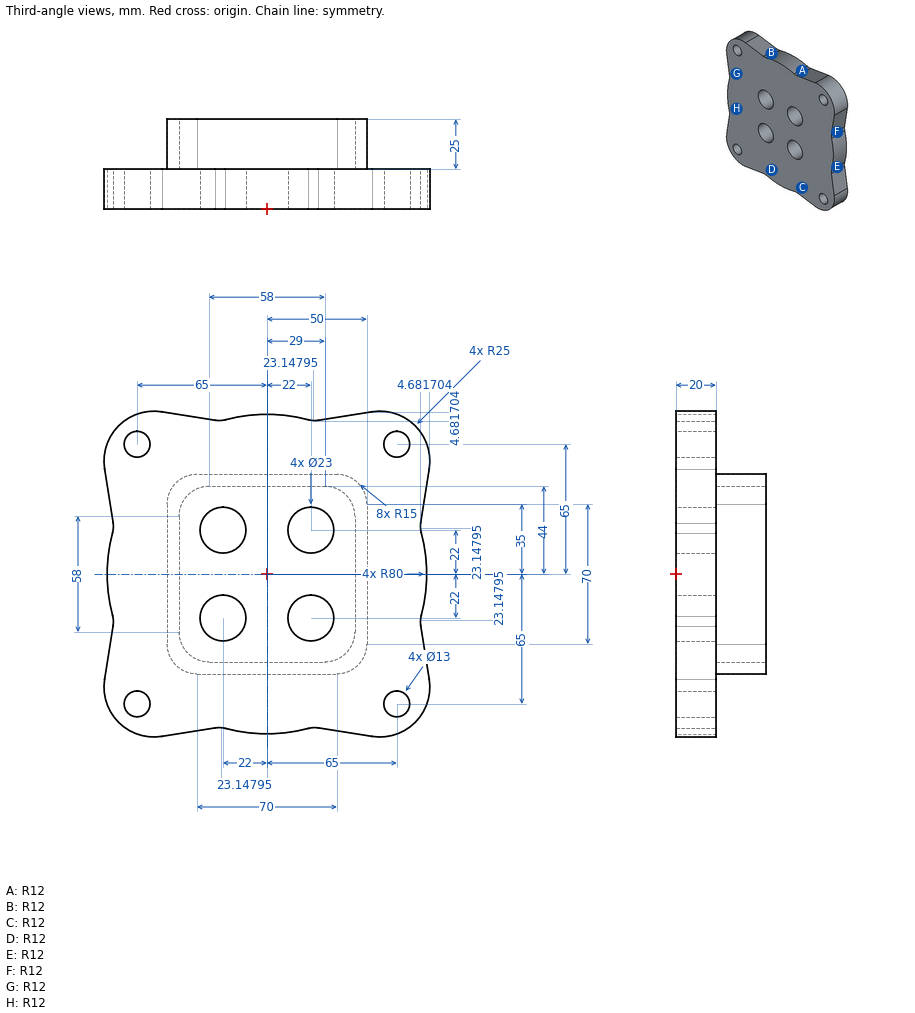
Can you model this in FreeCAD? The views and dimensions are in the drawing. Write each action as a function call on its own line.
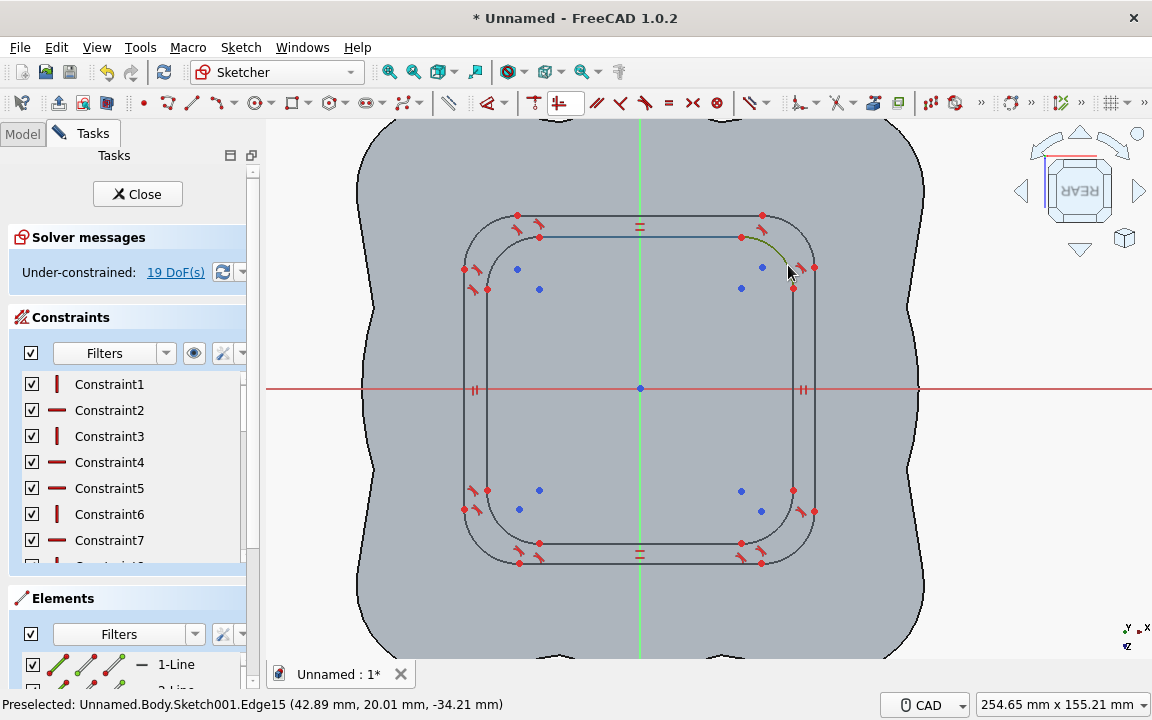
click(646, 104)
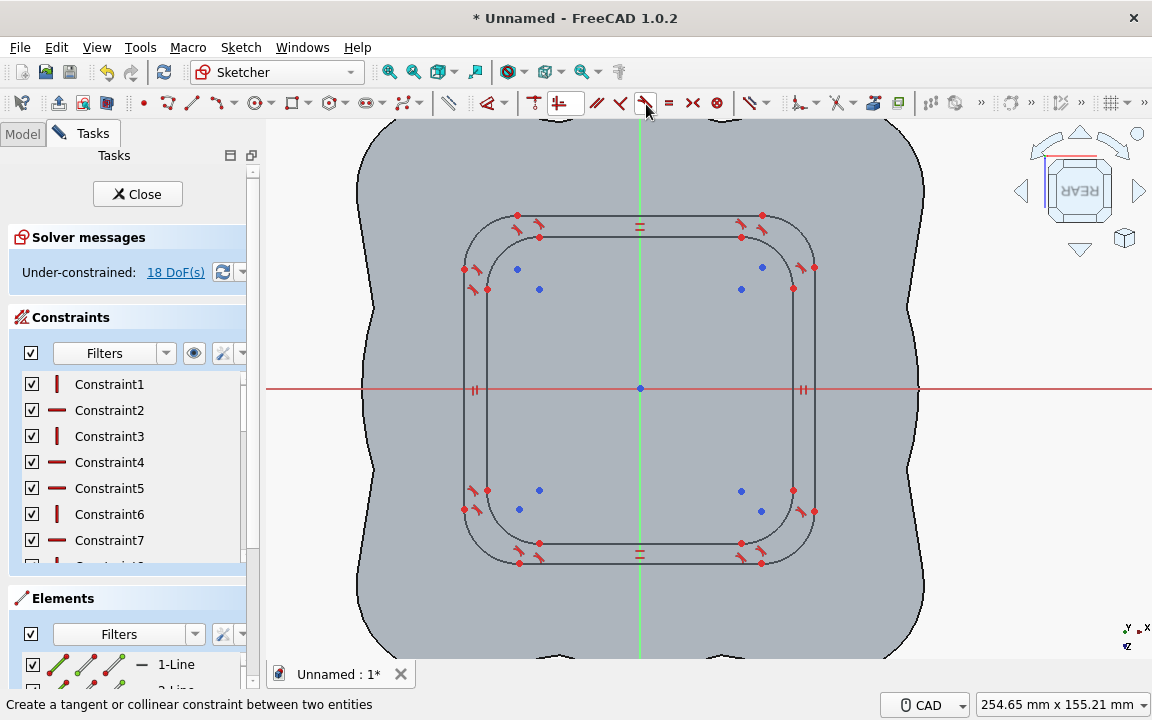
click(793, 350)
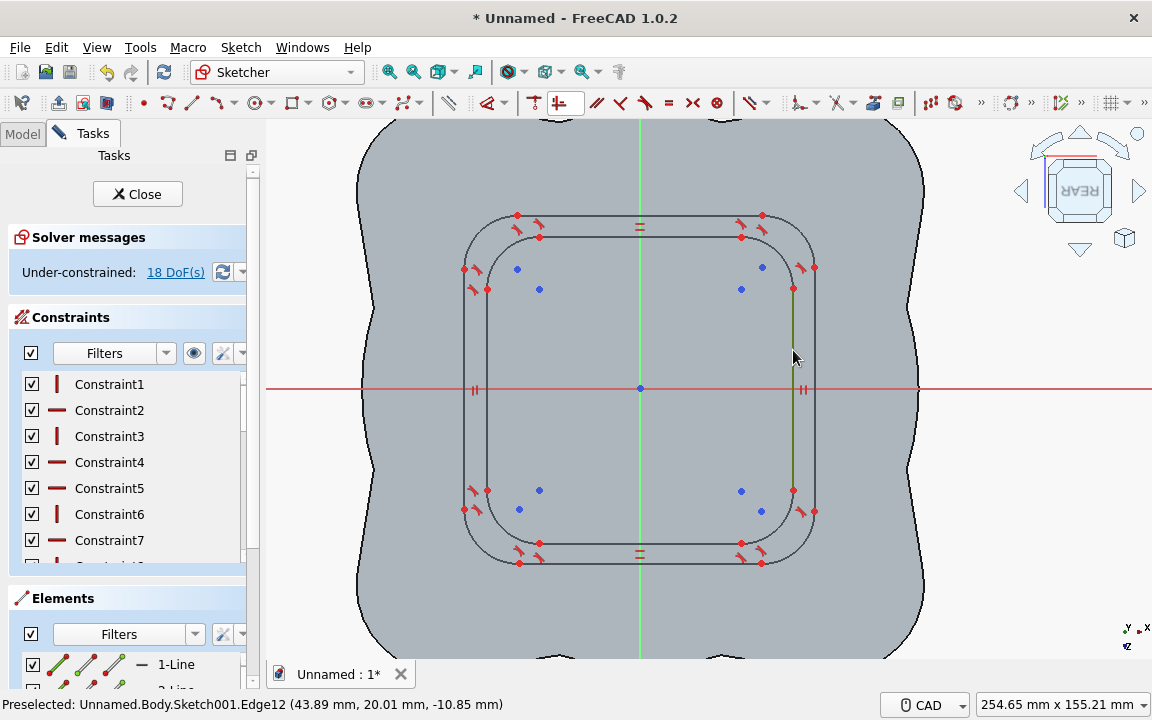
click(787, 265)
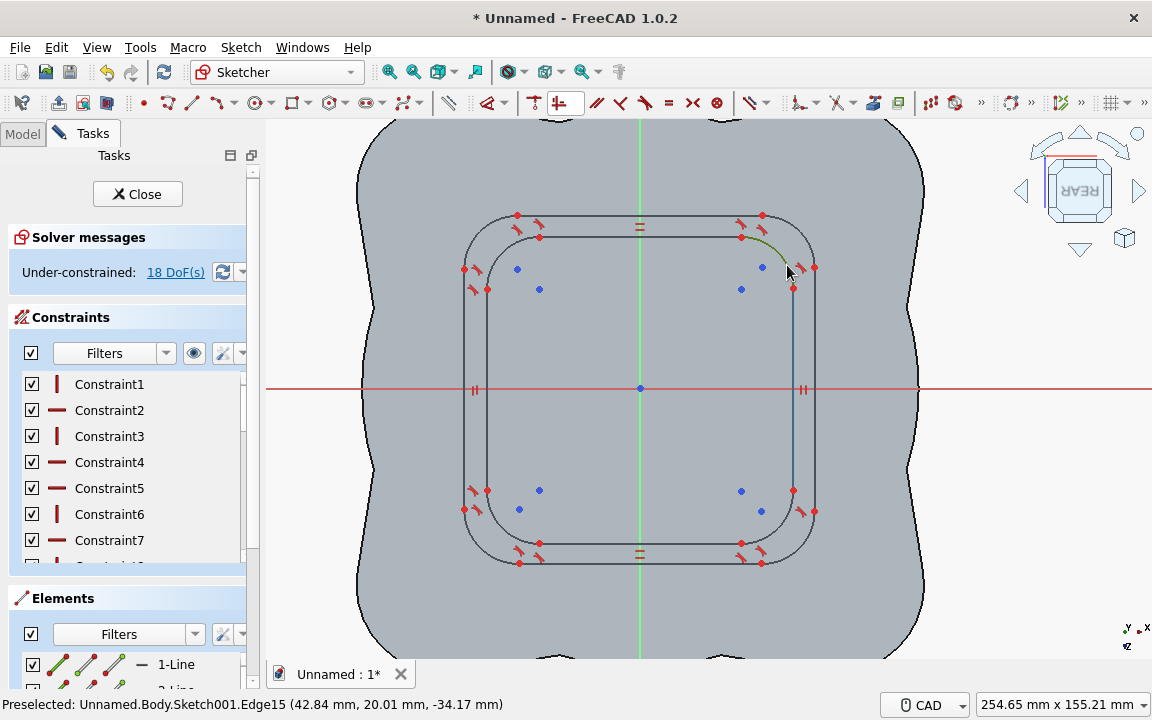
click(646, 104)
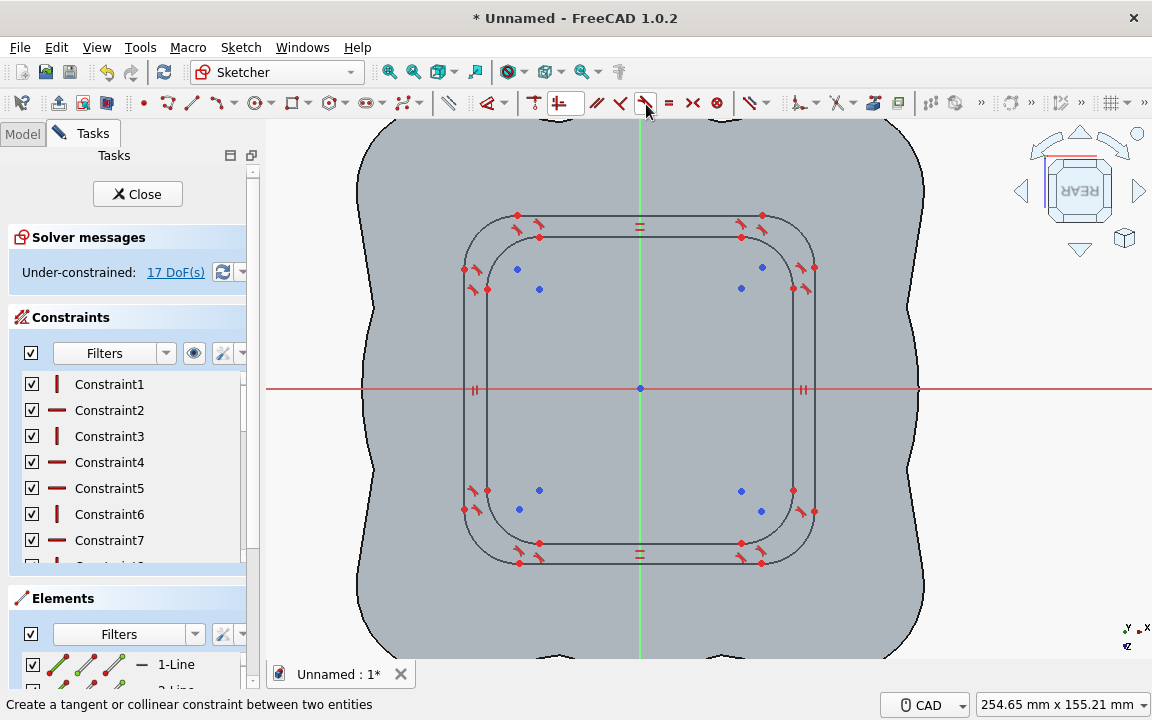
click(793, 350)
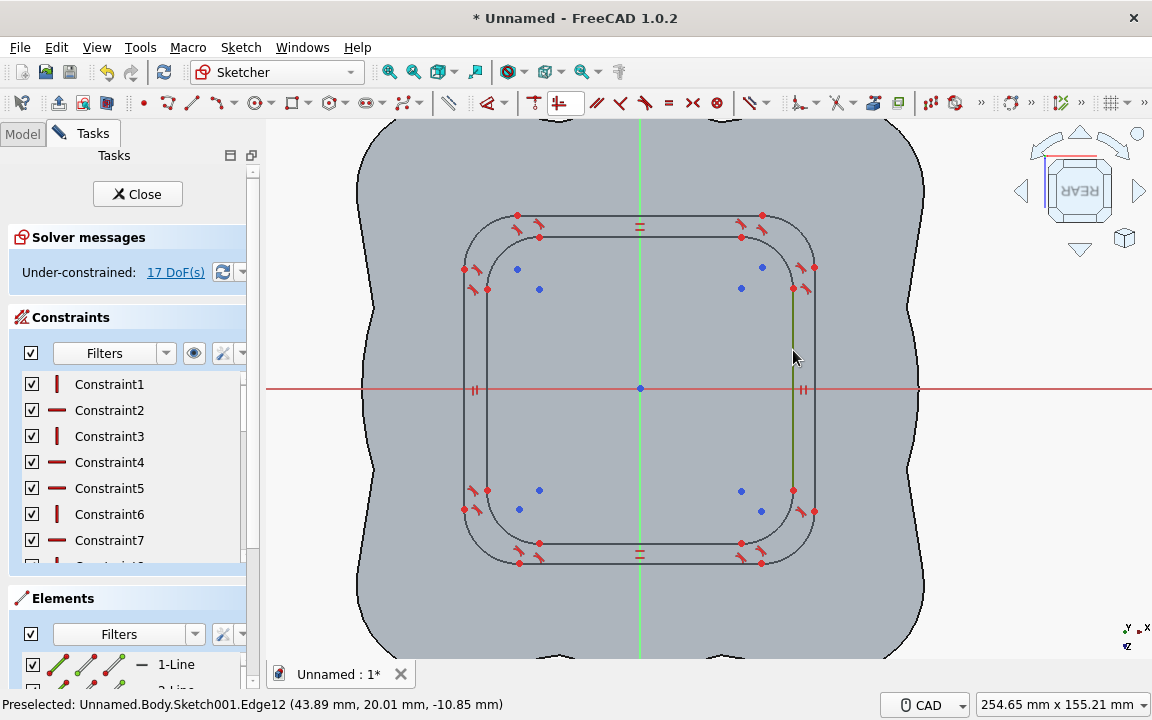
click(765, 538)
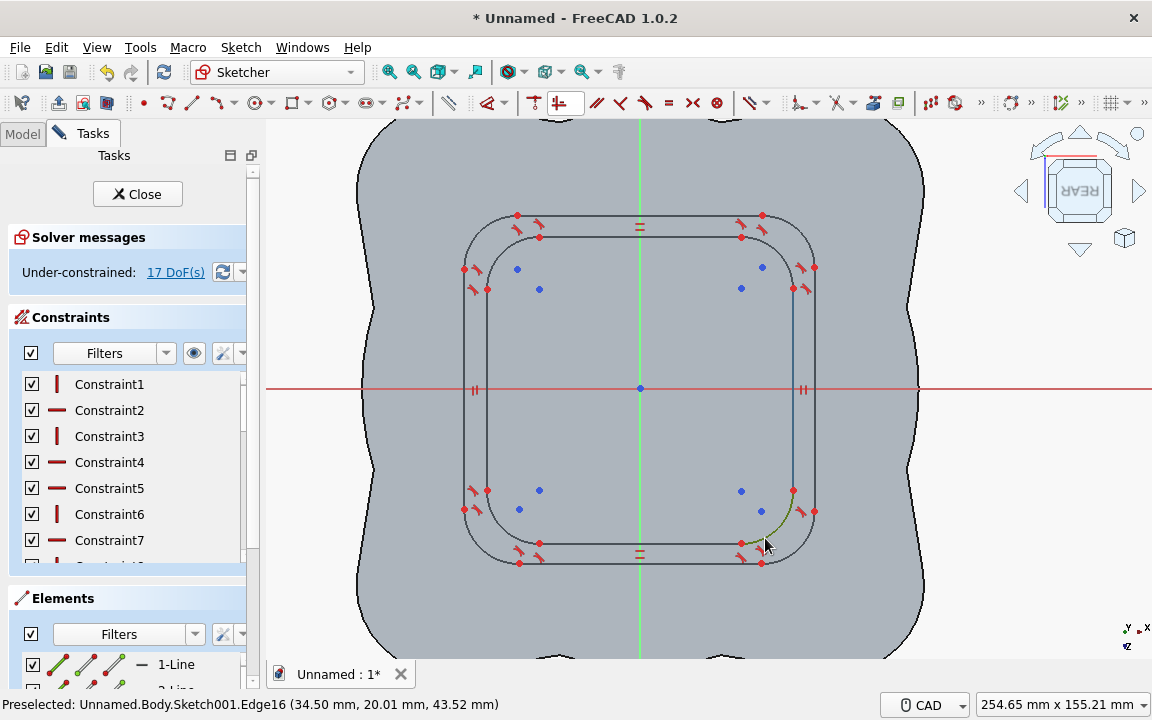
click(646, 104)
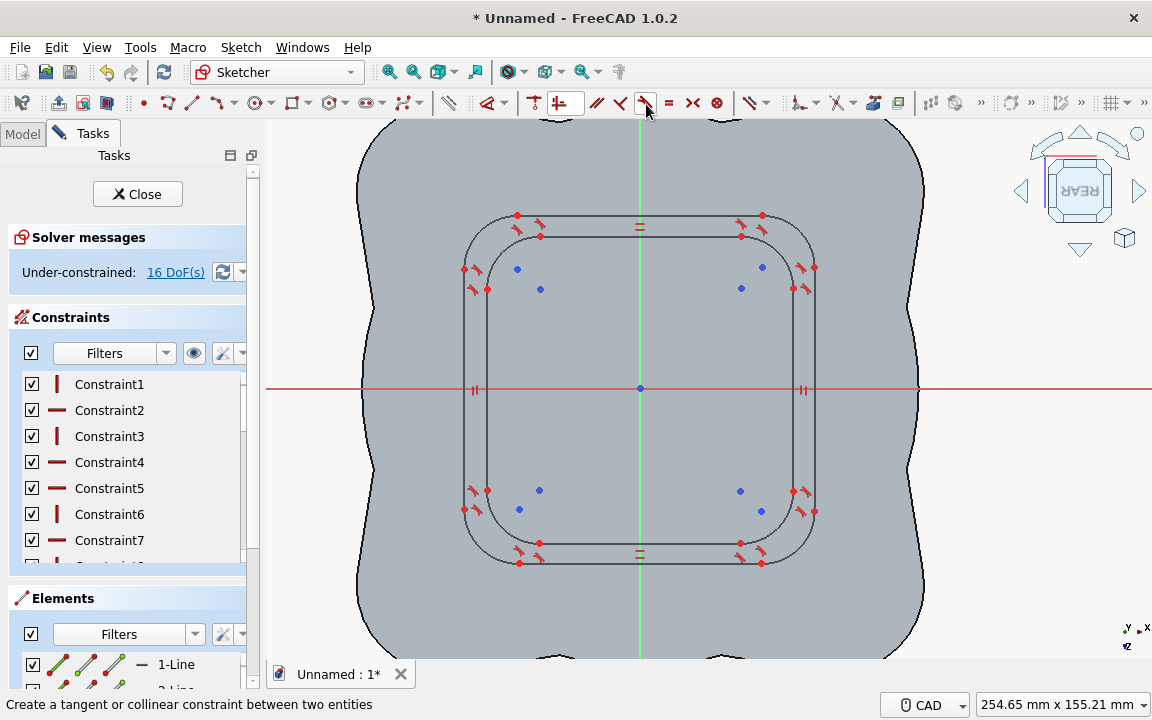
click(809, 244)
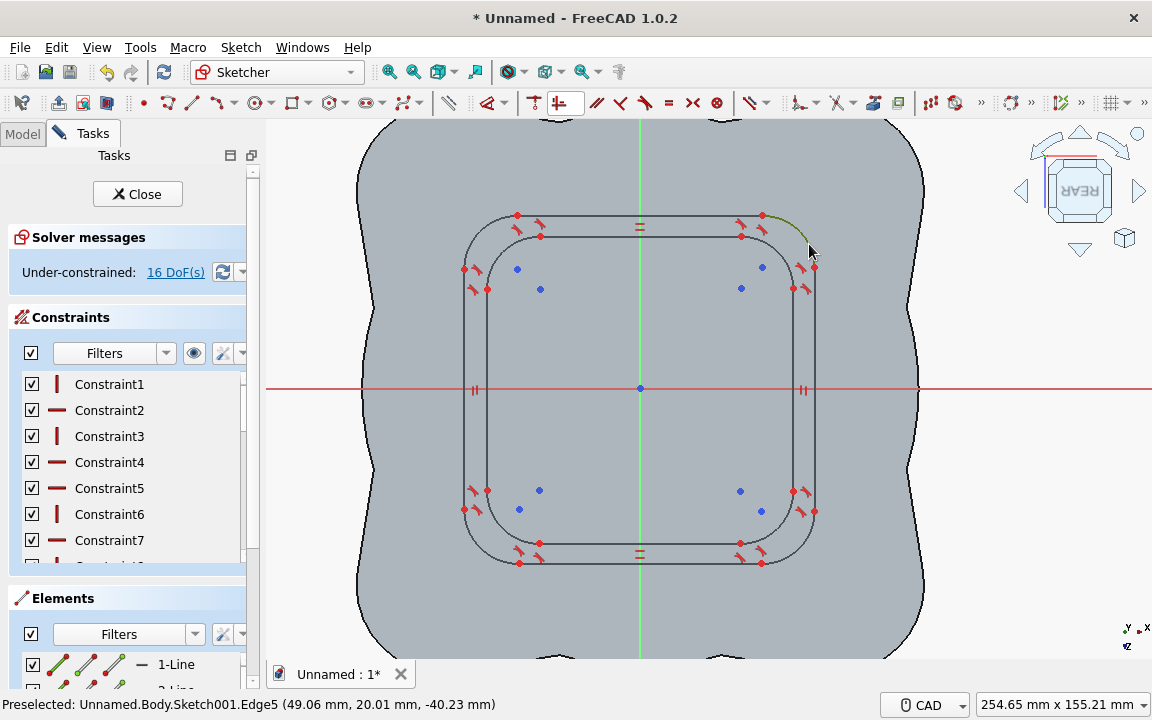
click(494, 222)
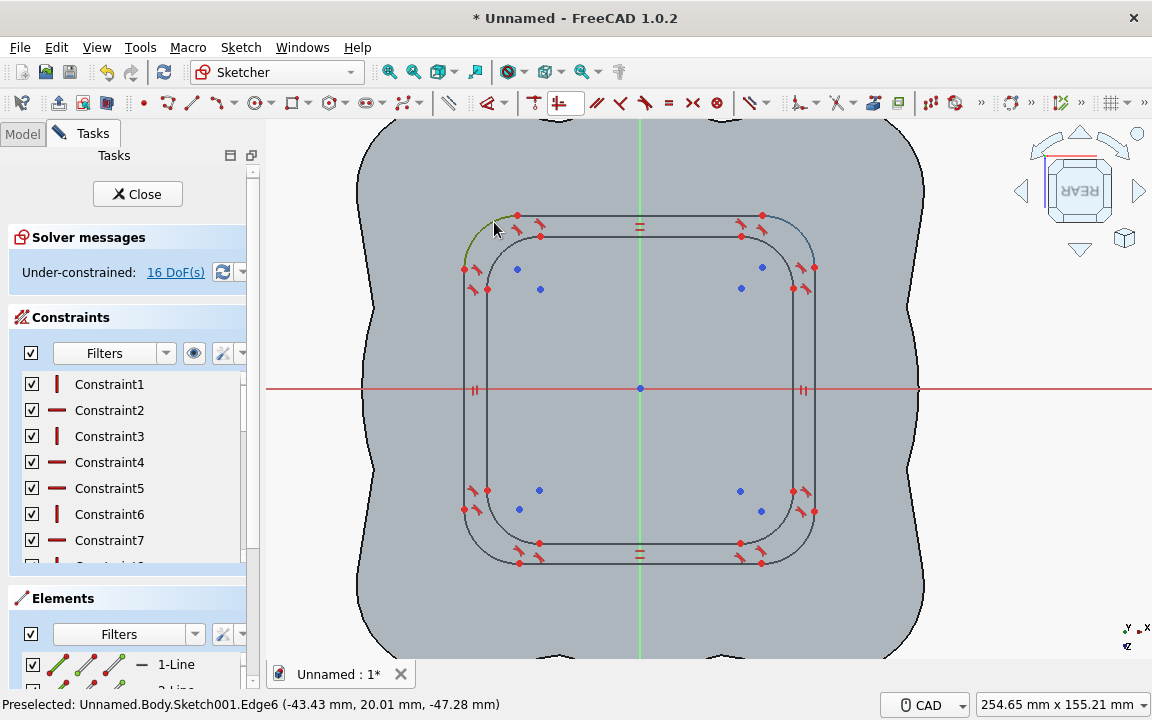
click(470, 534)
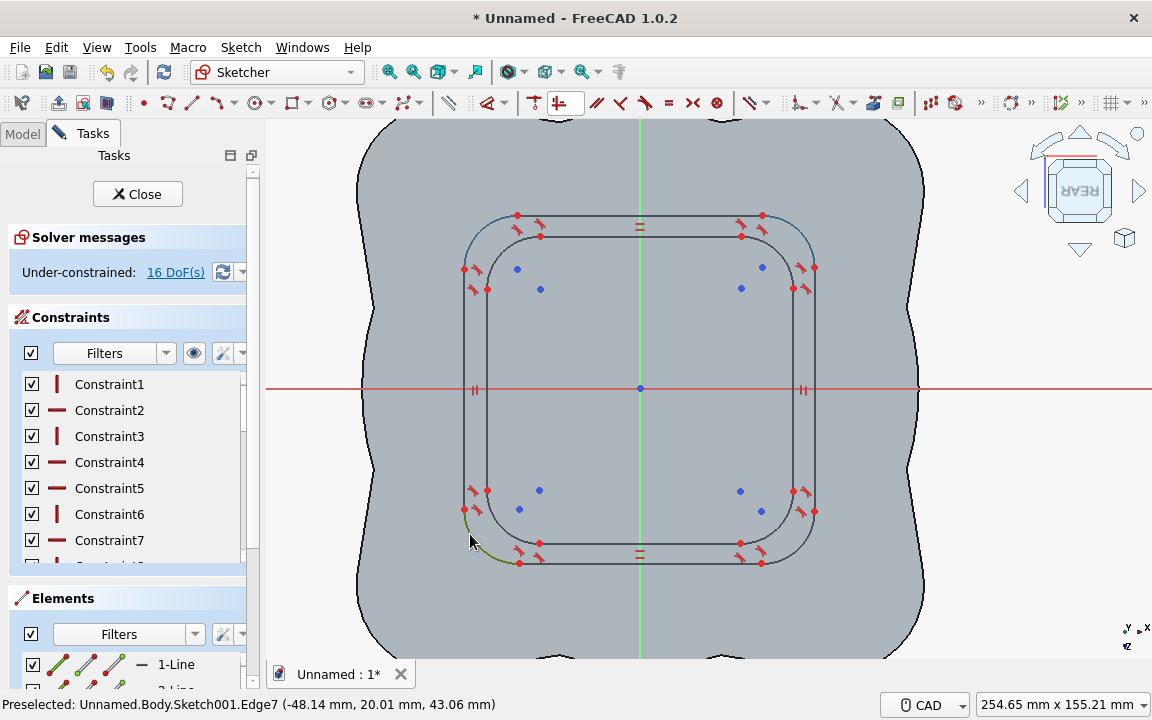
click(786, 558)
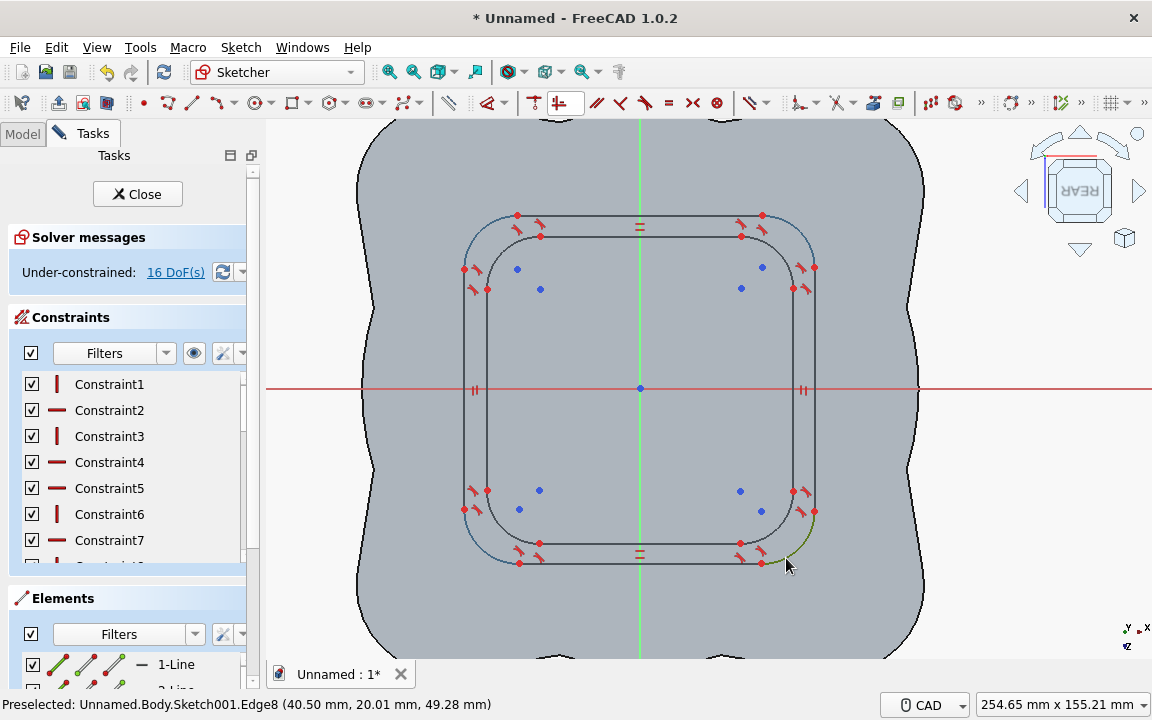
click(493, 515)